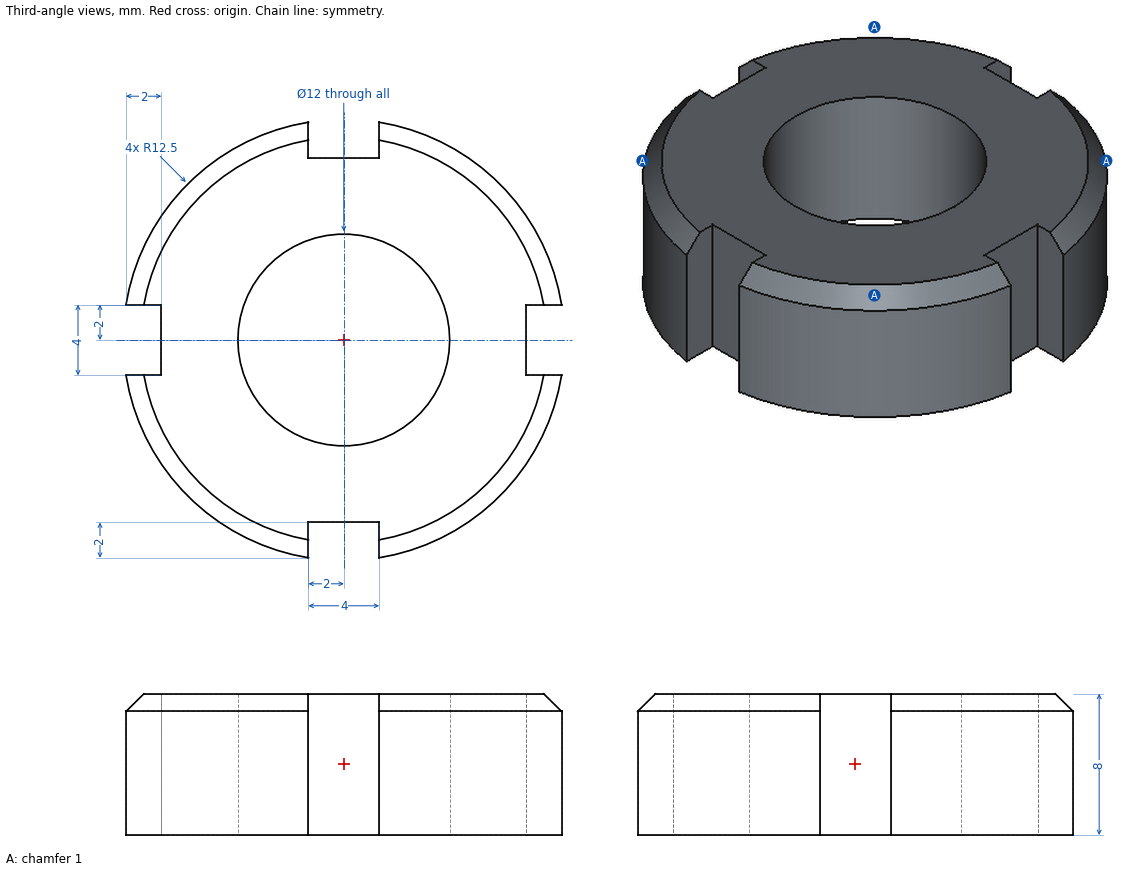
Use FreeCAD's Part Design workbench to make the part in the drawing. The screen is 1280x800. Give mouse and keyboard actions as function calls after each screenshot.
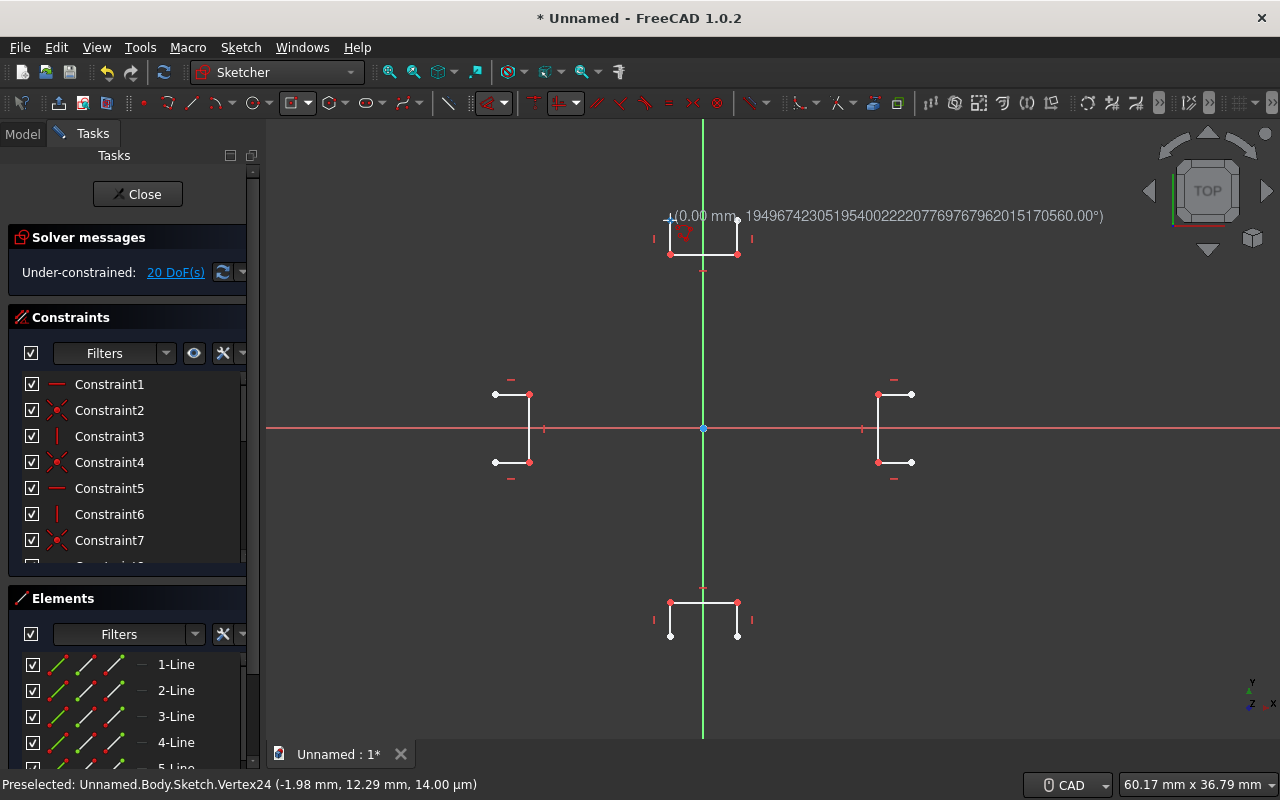
key(g)
key(3)
key(a)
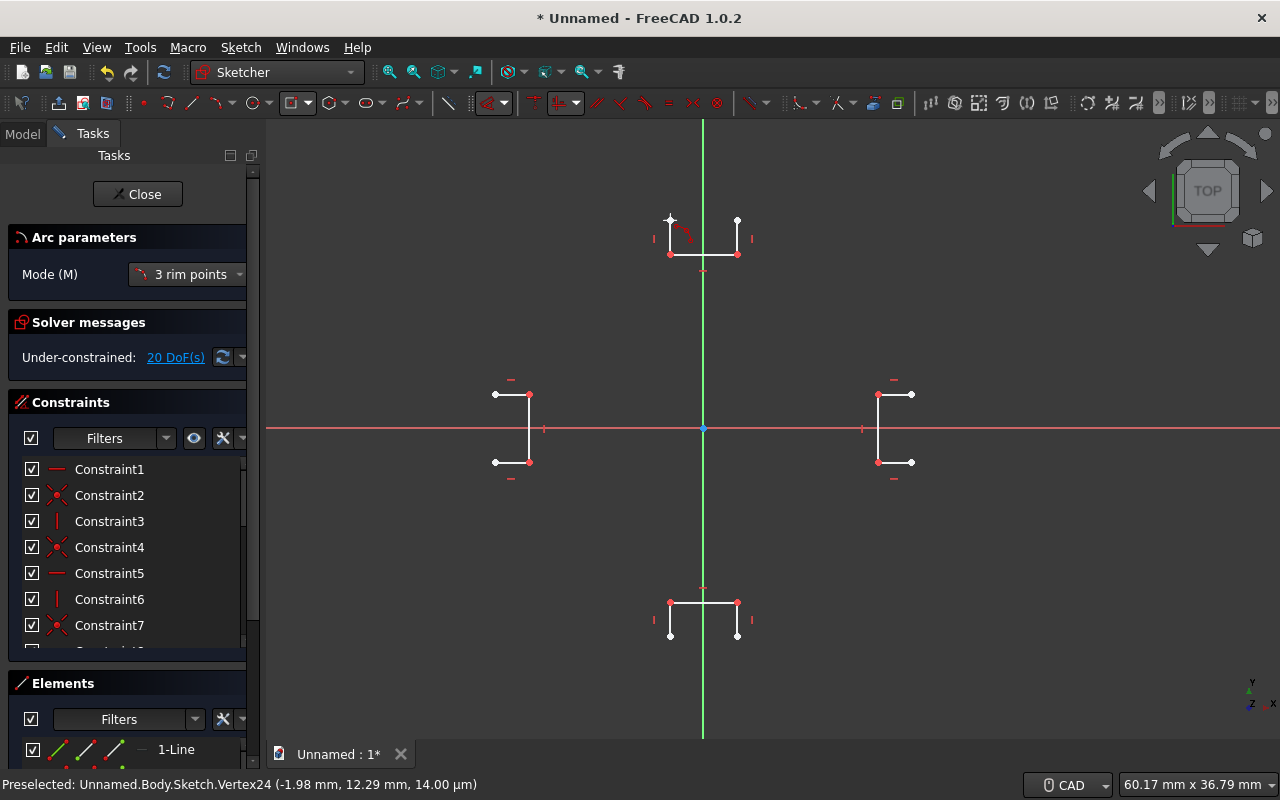
click(495, 463)
click(670, 637)
click(554, 577)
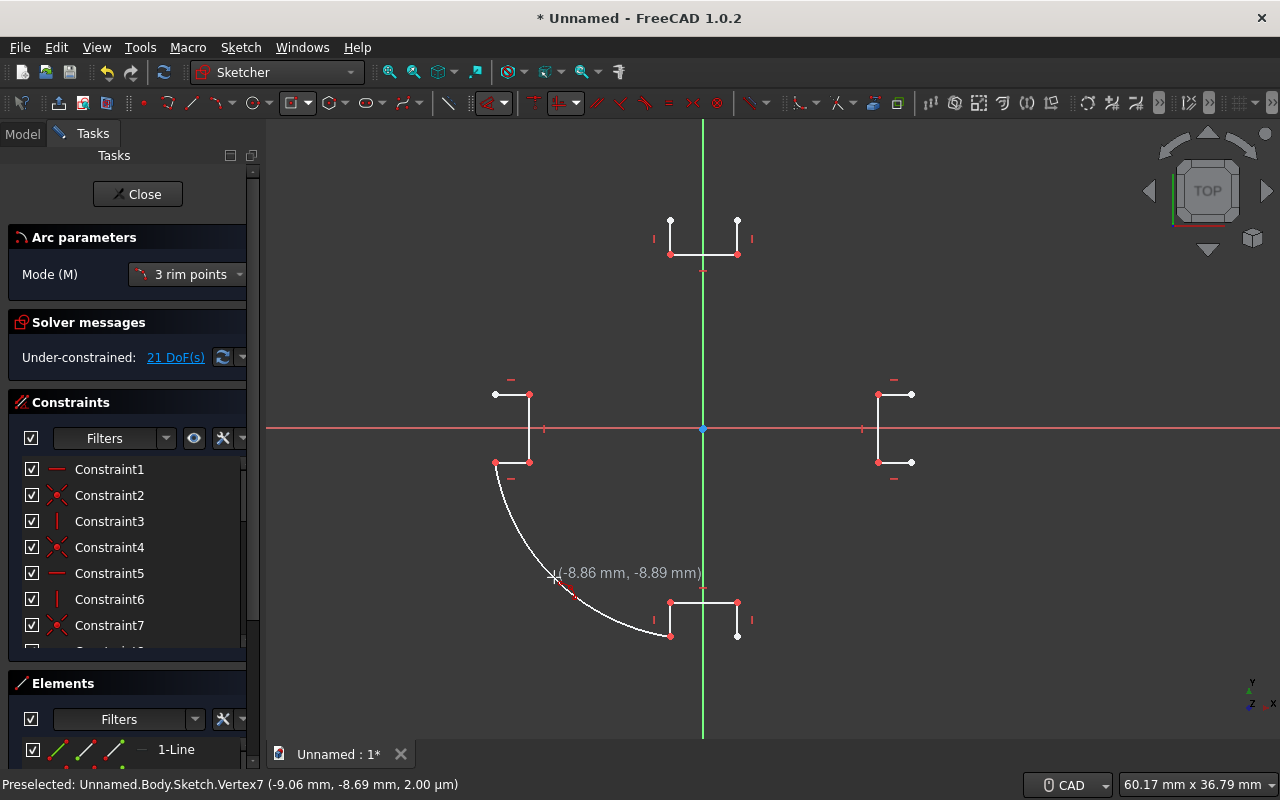
click(737, 637)
click(911, 463)
click(852, 577)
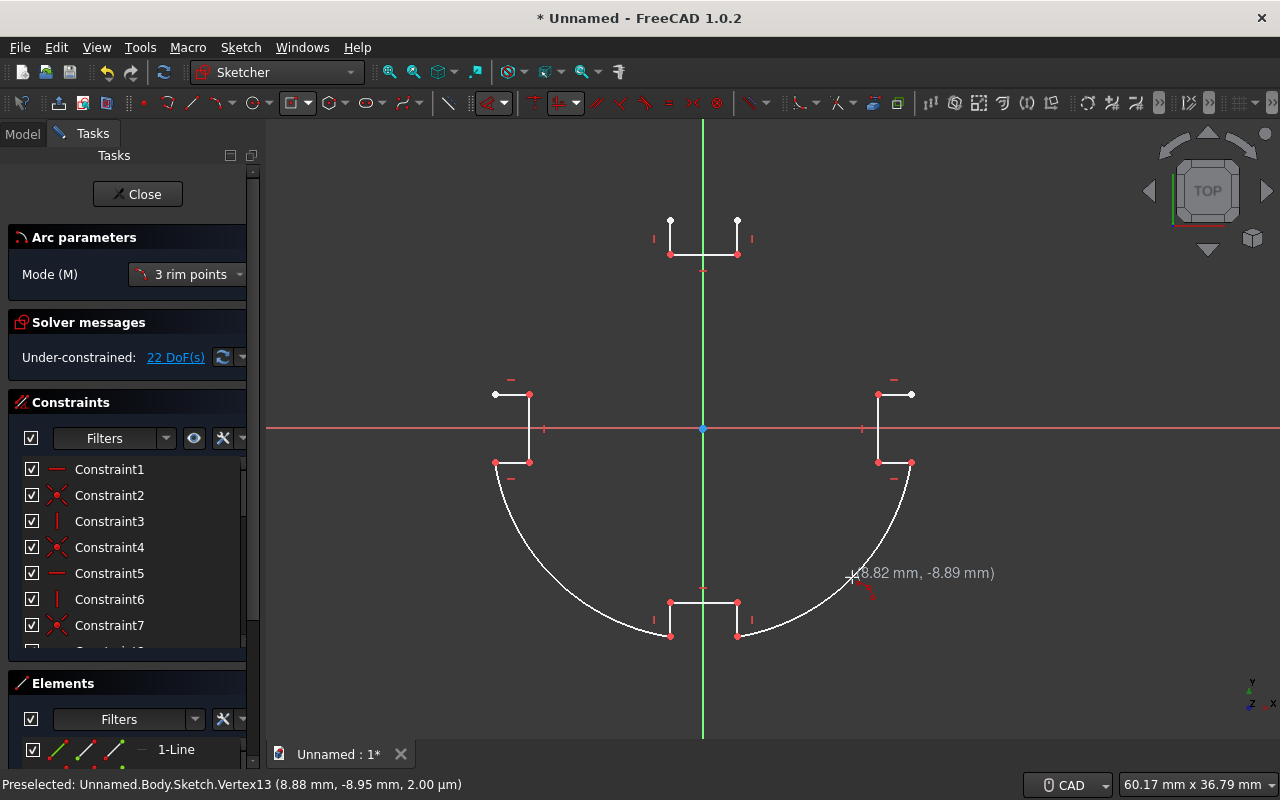
click(911, 395)
click(737, 221)
click(852, 279)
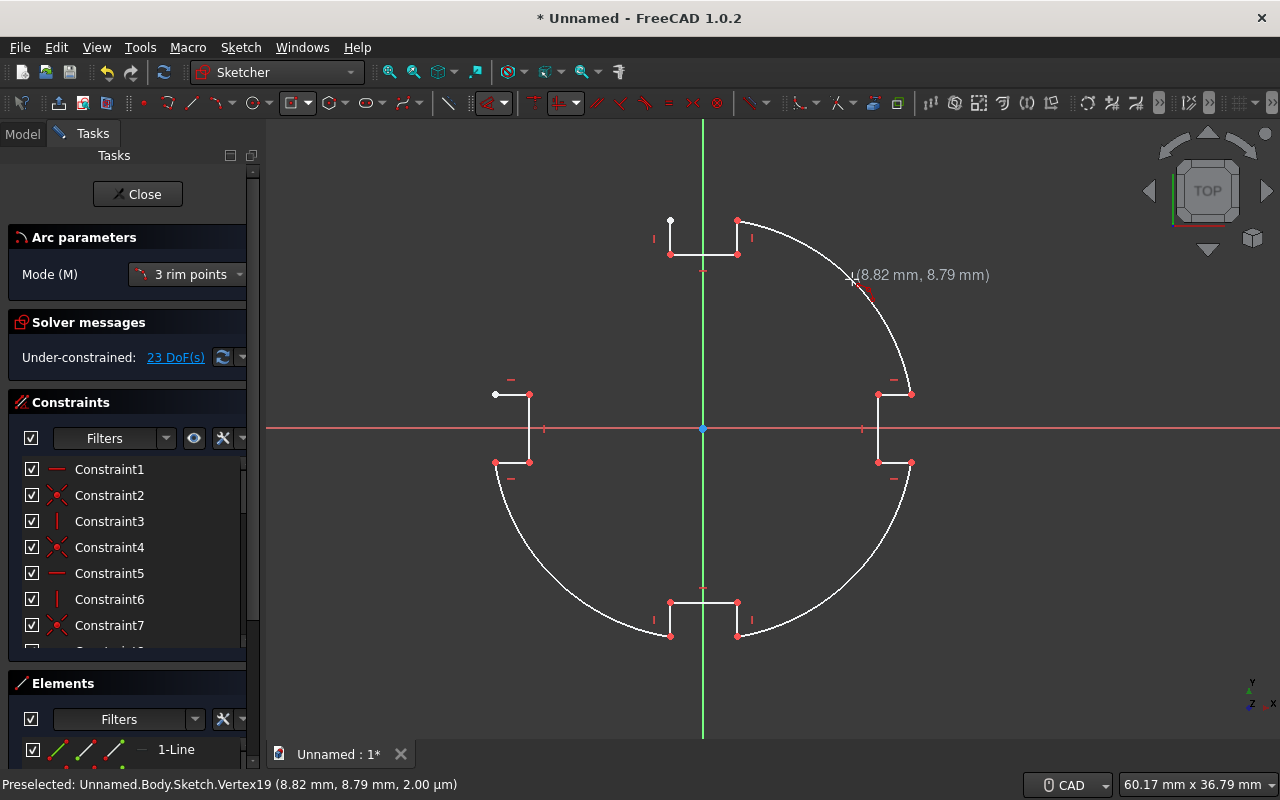
click(670, 221)
click(495, 395)
click(554, 279)
key(Escape)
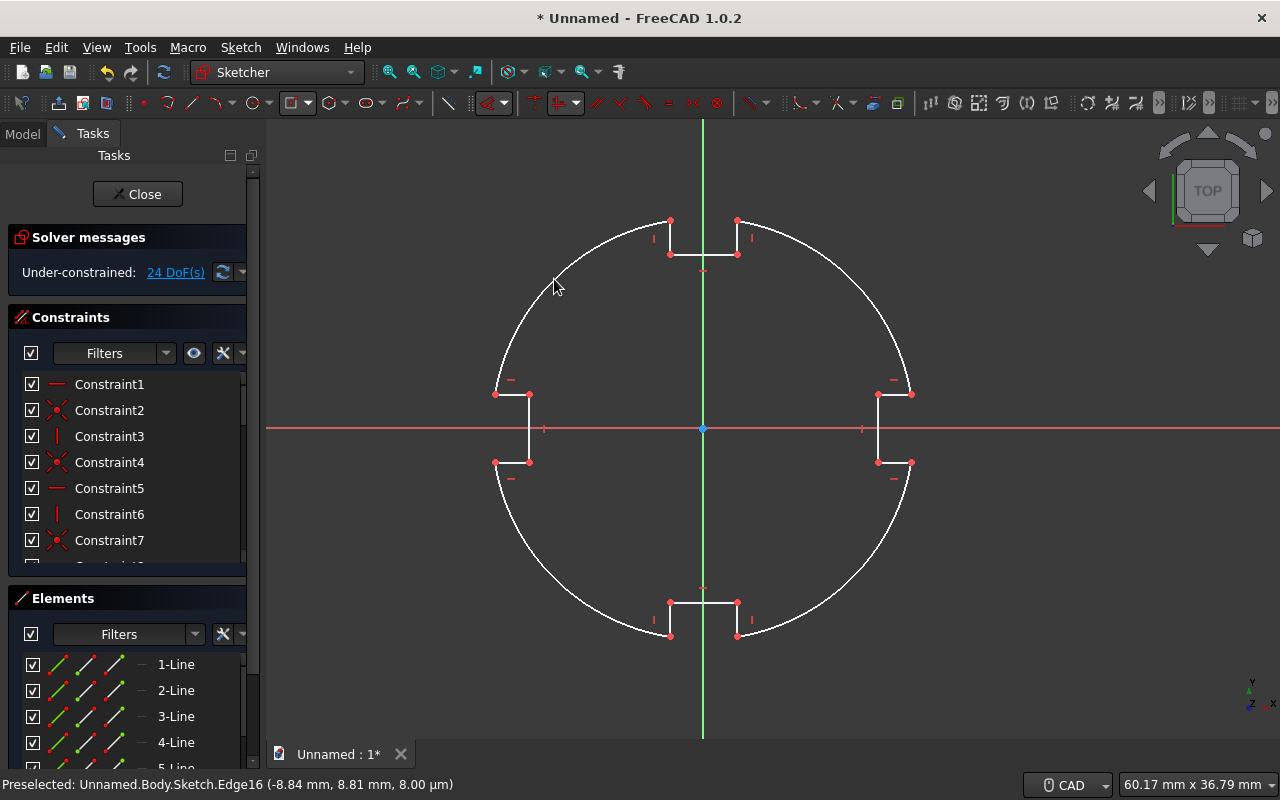
click(522, 537)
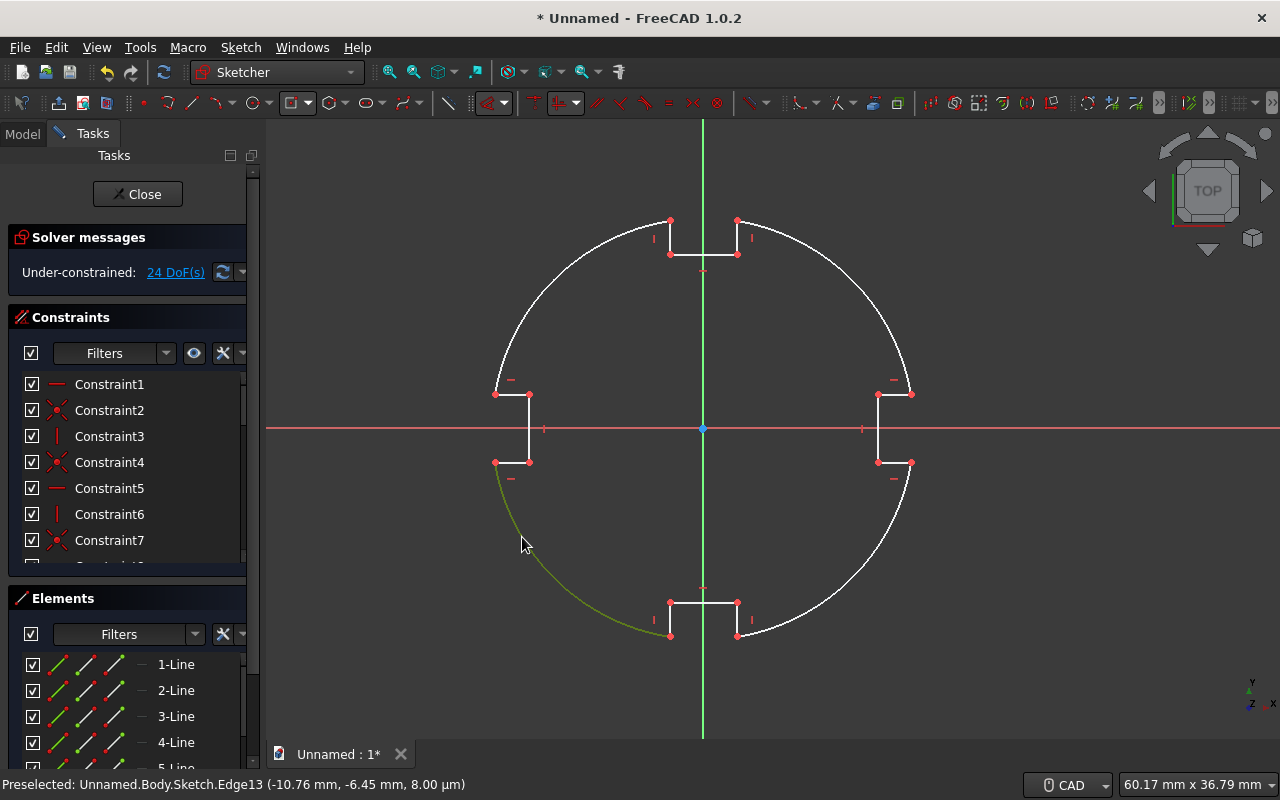
click(811, 610)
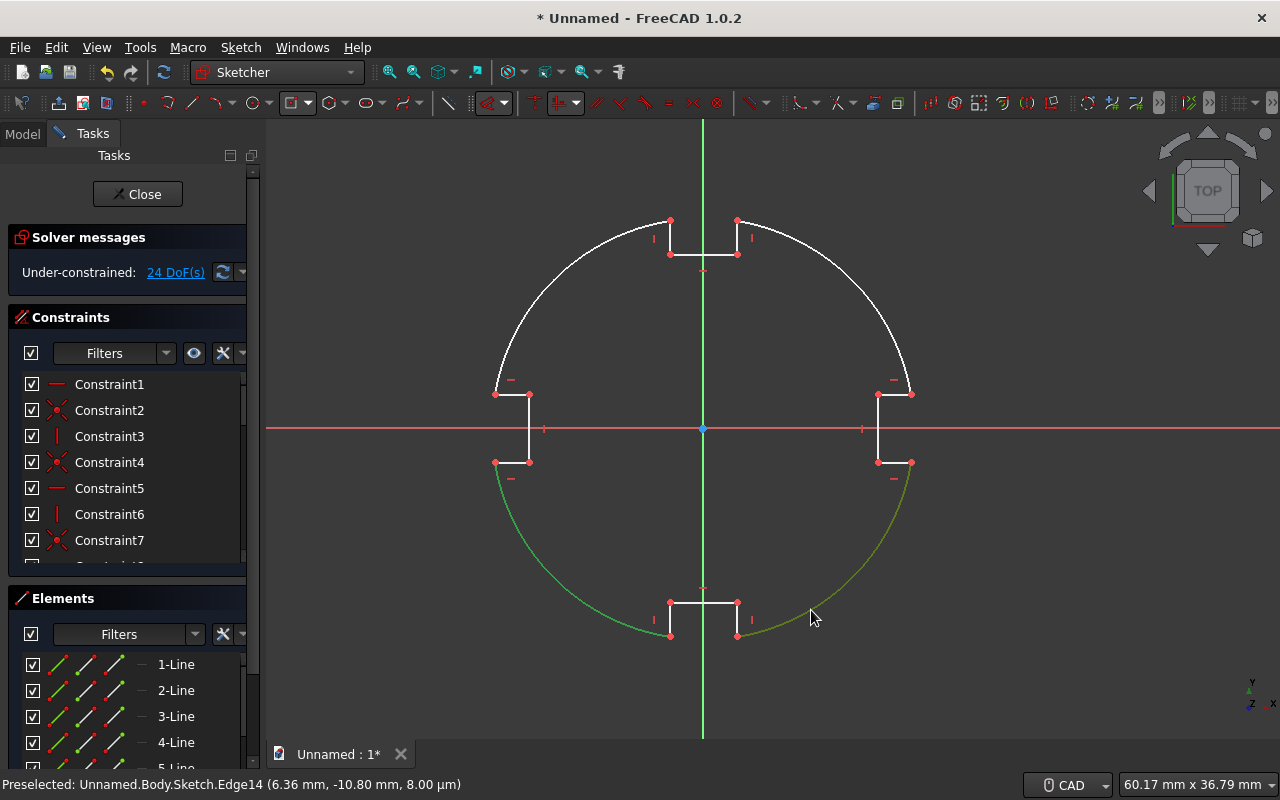
key(c)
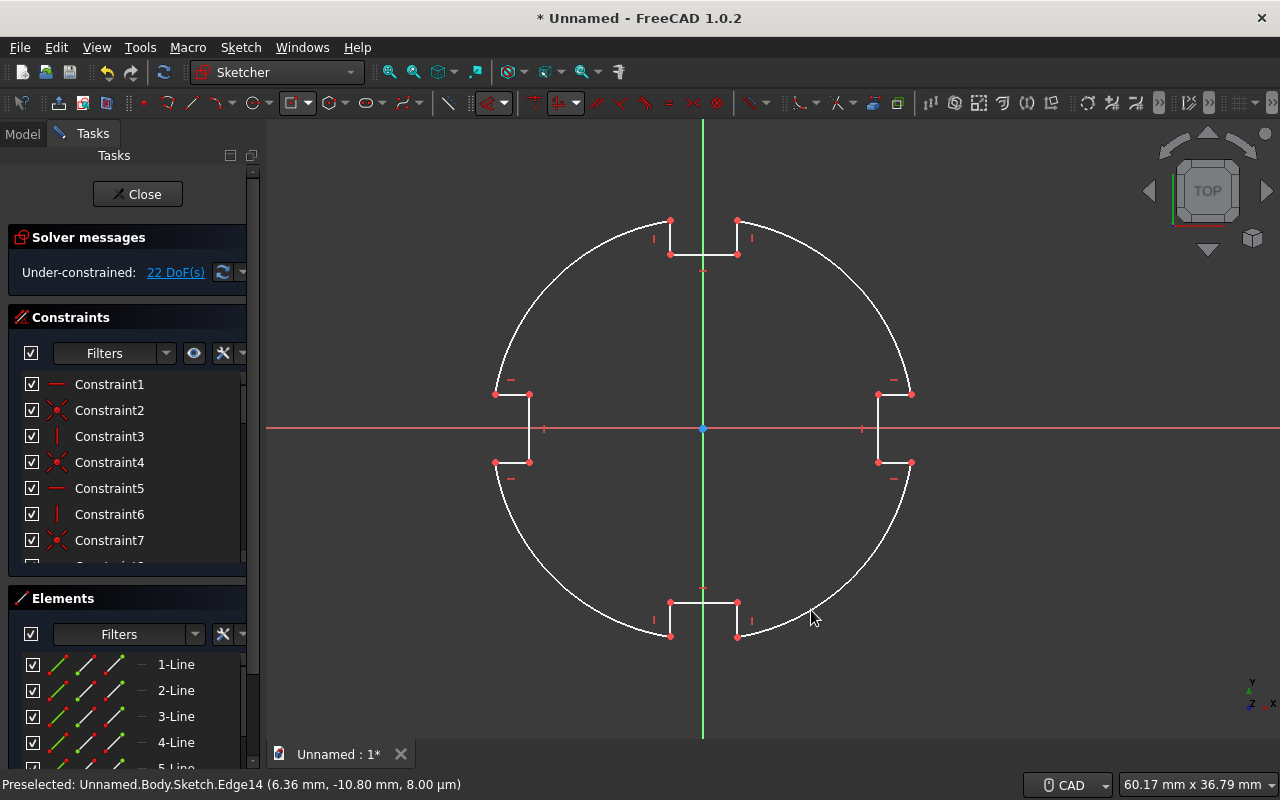
click(522, 537)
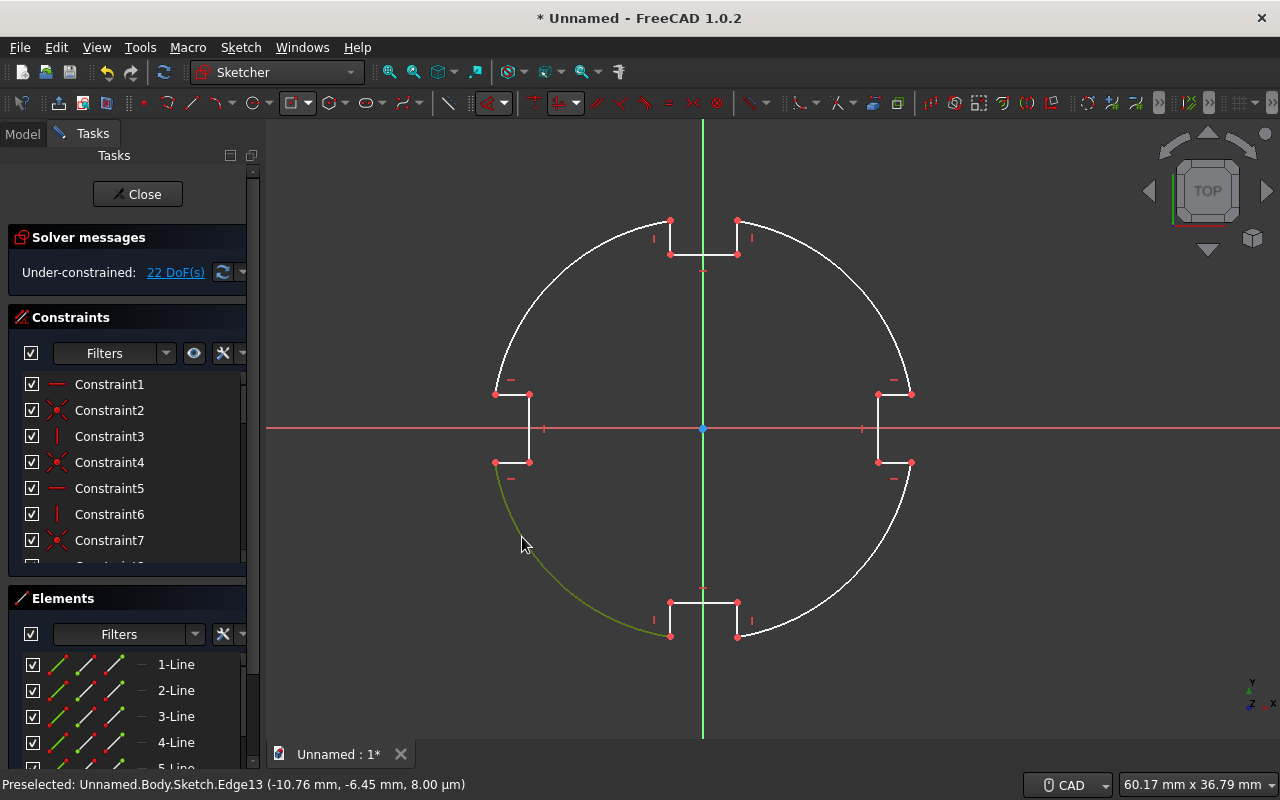
click(884, 321)